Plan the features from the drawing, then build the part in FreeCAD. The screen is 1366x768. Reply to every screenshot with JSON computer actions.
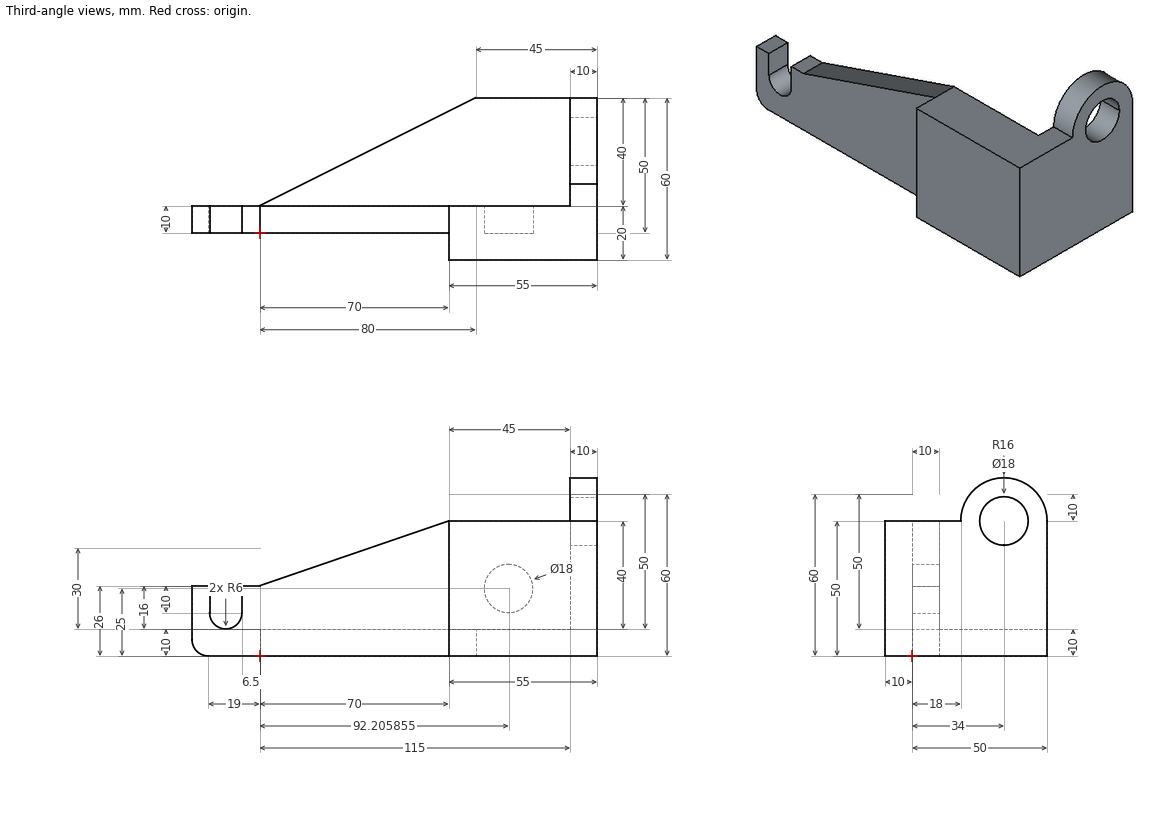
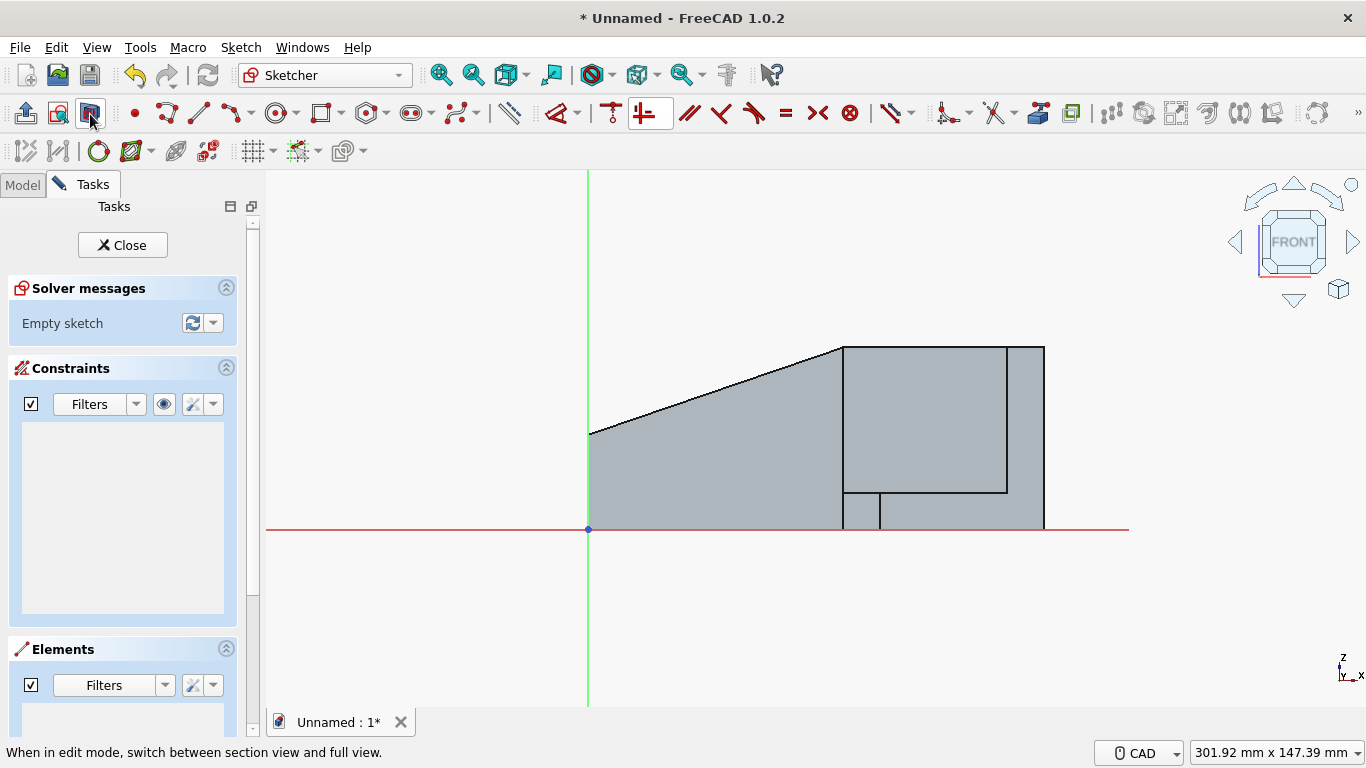
{"action": "scroll", "coordinate": [455, 501], "scroll_direction": "up", "scroll_amount": 6}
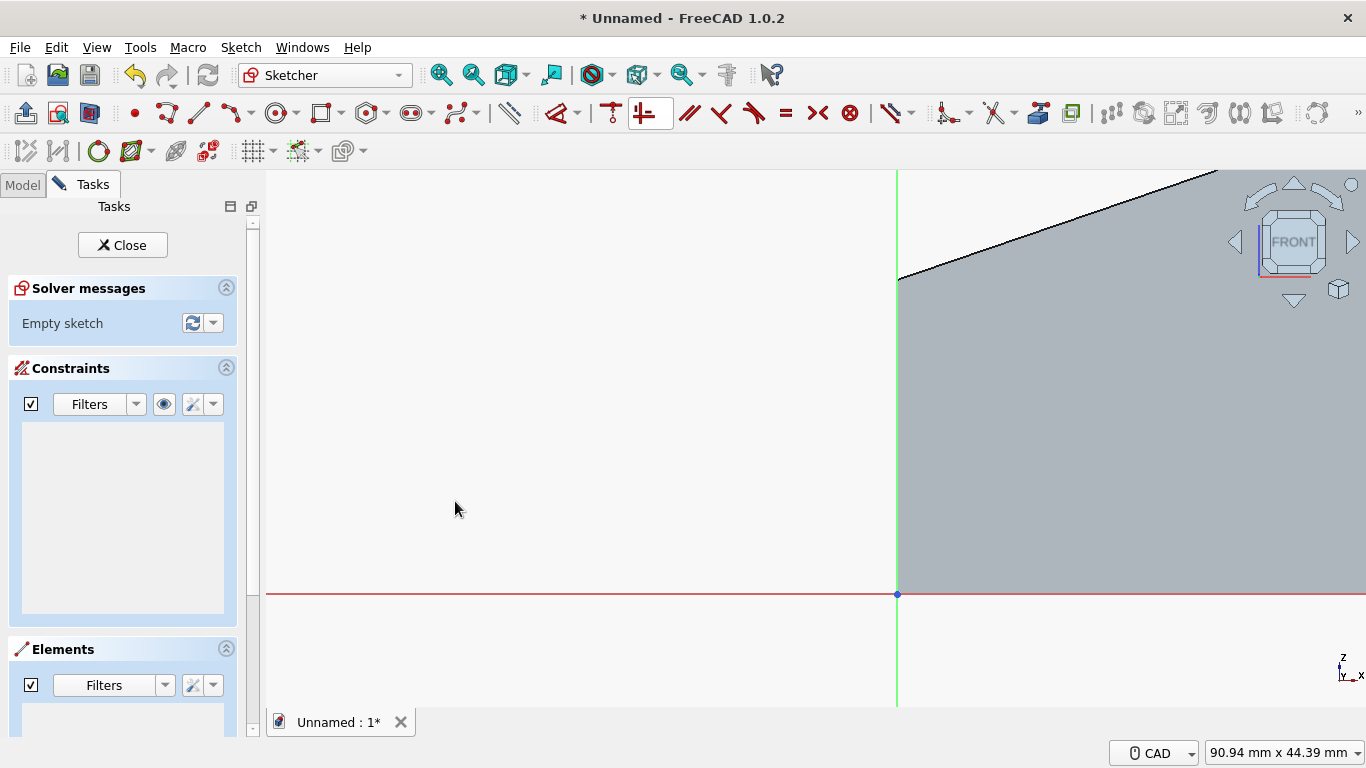
{"action": "left_click", "coordinate": [168, 114]}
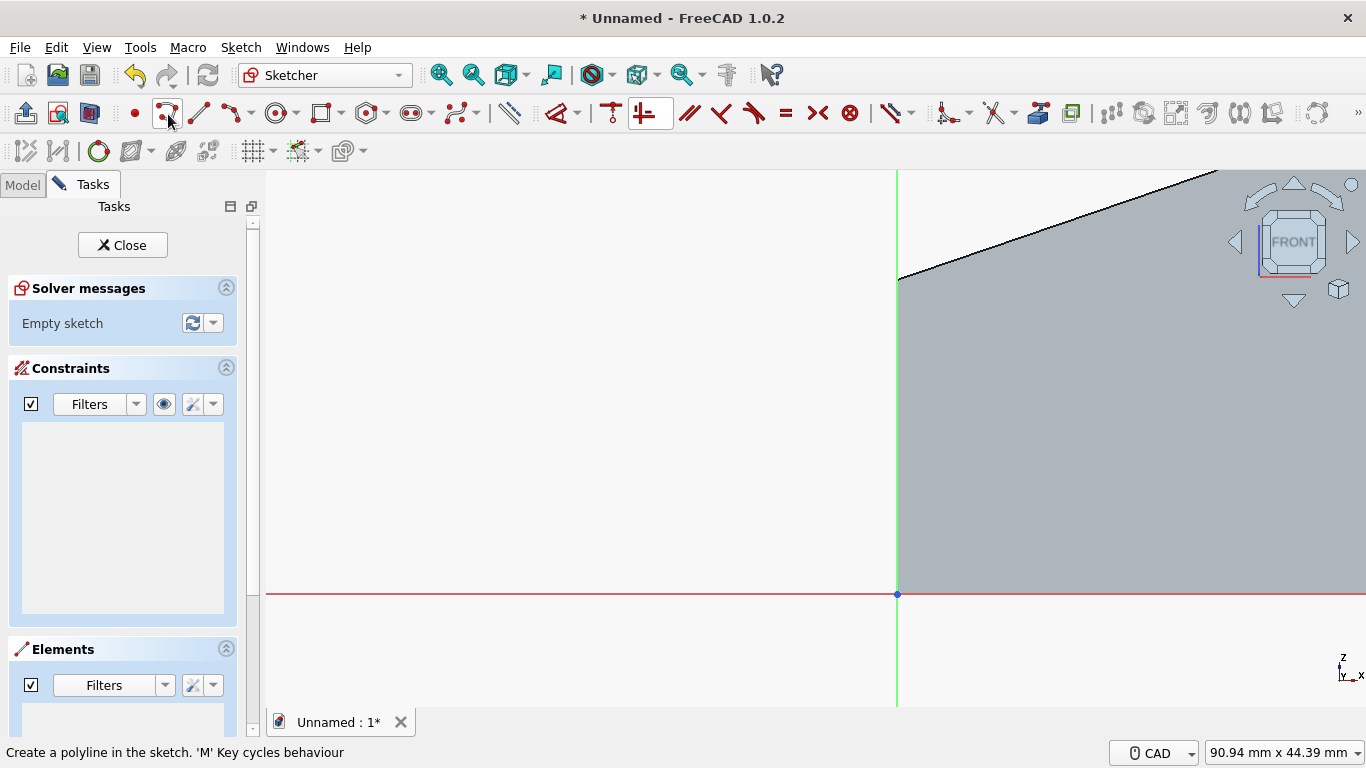
{"action": "left_click", "coordinate": [667, 594]}
{"action": "left_click", "coordinate": [897, 594]}
{"action": "left_click", "coordinate": [888, 280]}
{"action": "left_click", "coordinate": [819, 280]}
{"action": "left_click", "coordinate": [819, 401]}
{"action": "right_click", "coordinate": [819, 401]}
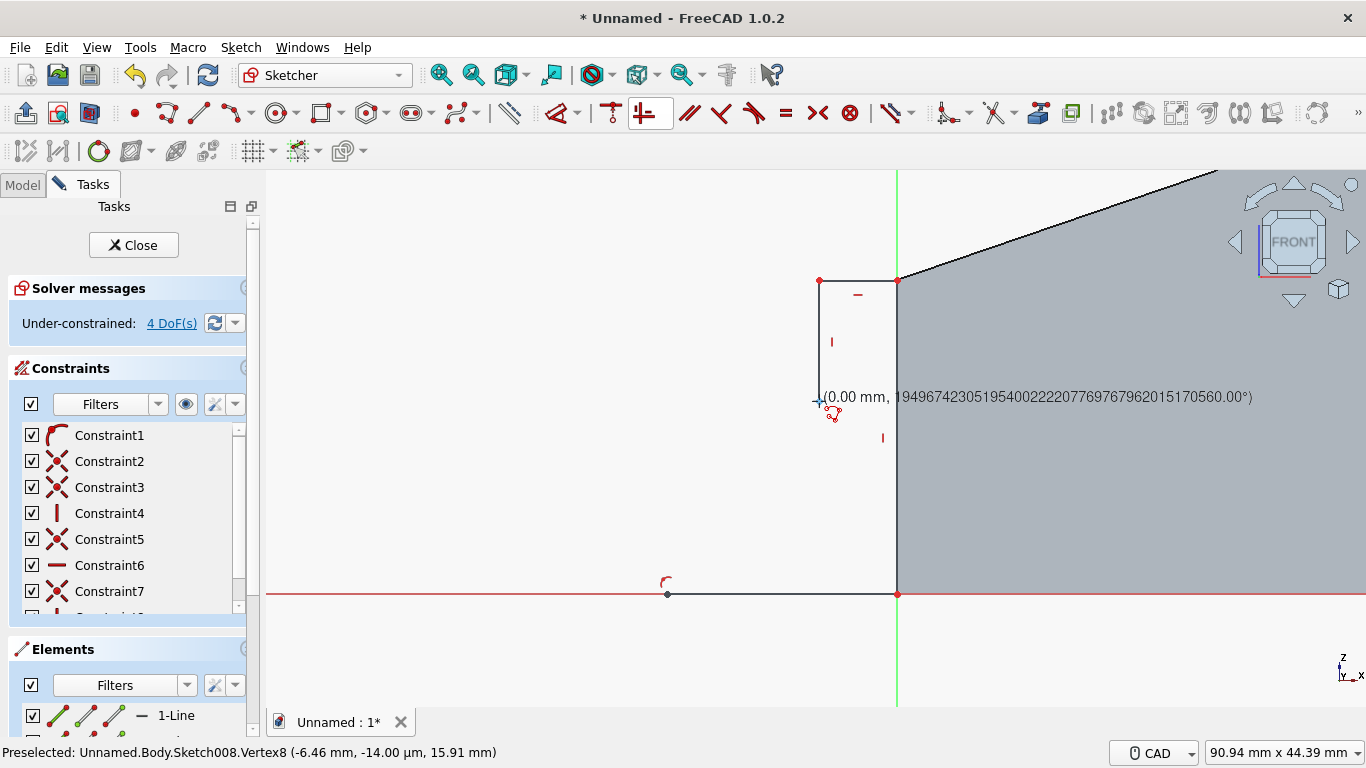
{"action": "left_click", "coordinate": [673, 401]}
{"action": "left_click", "coordinate": [673, 280]}
{"action": "left_click", "coordinate": [595, 280]}
{"action": "left_click", "coordinate": [595, 522]}
{"action": "right_click", "coordinate": [595, 522]}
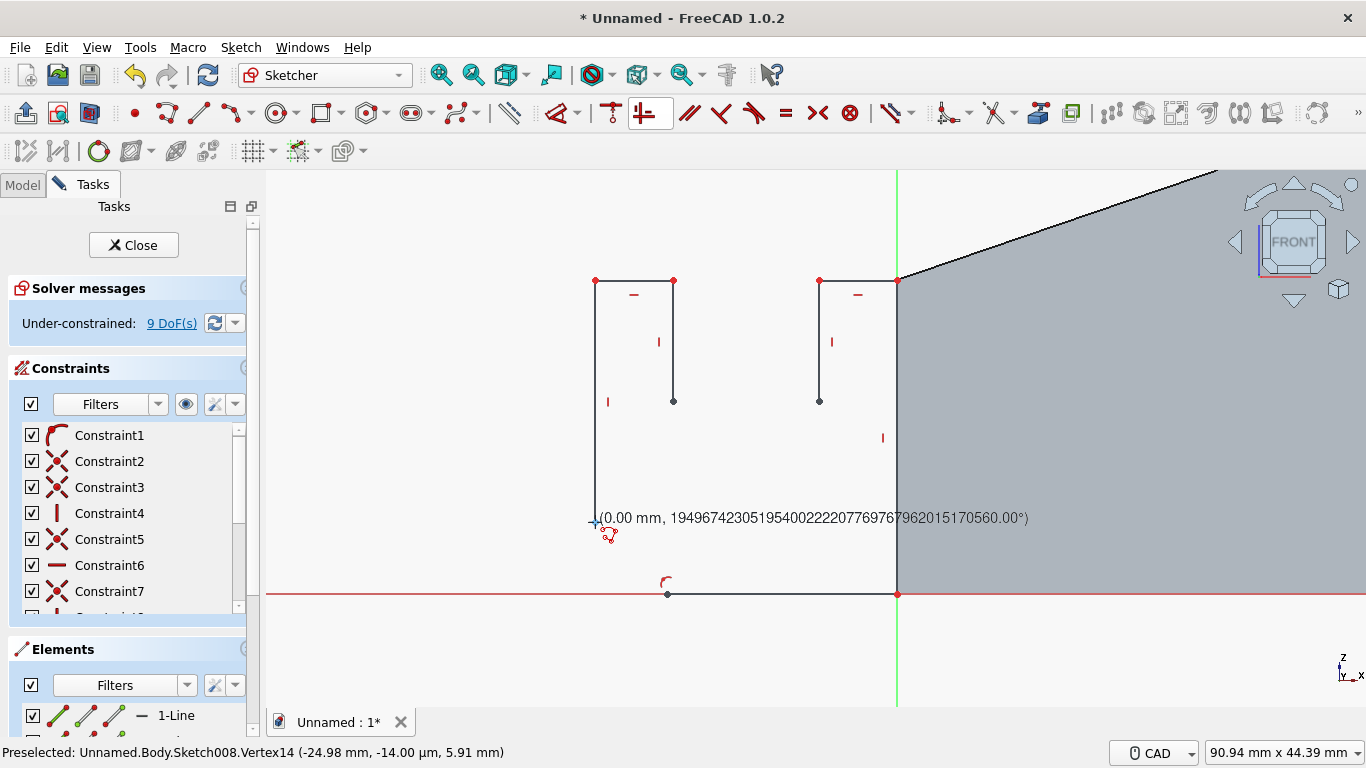
{"action": "left_click", "coordinate": [232, 114]}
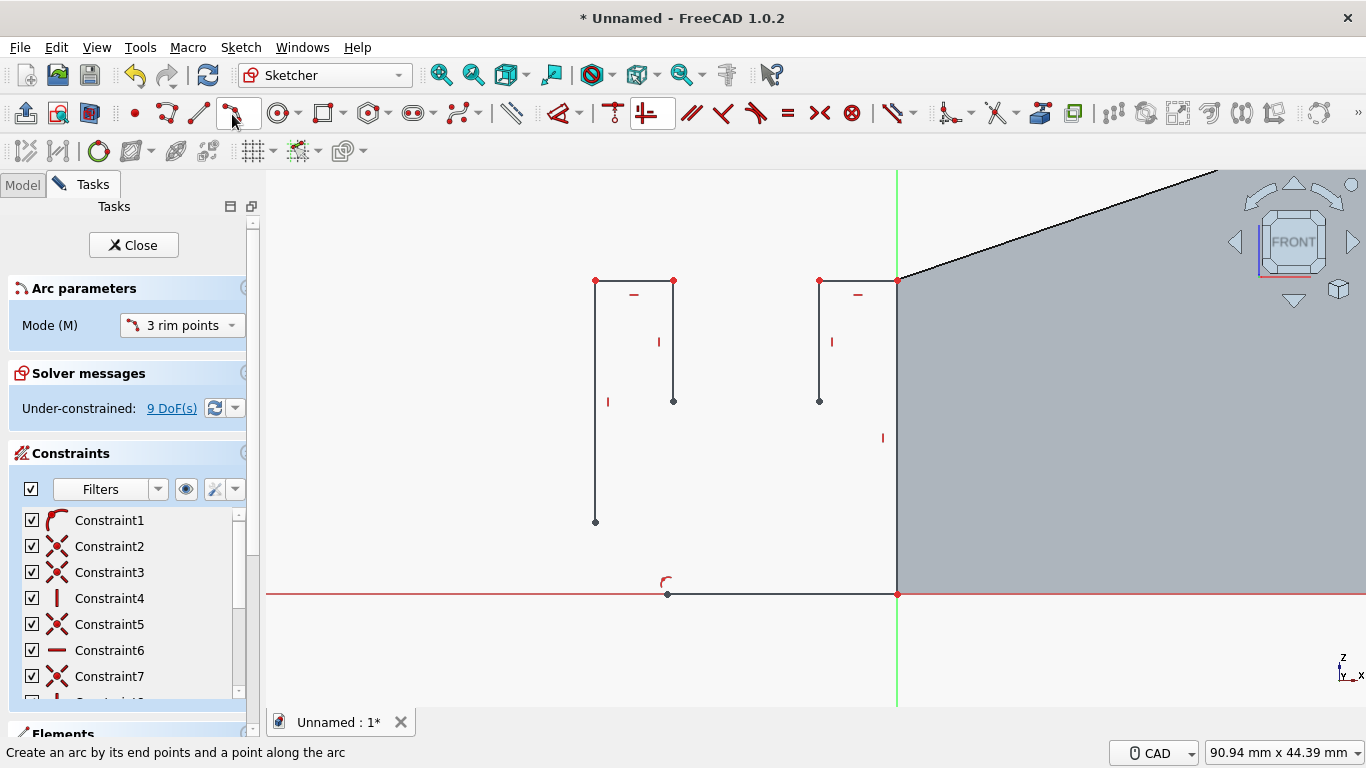
{"action": "left_click", "coordinate": [819, 402]}
{"action": "left_click", "coordinate": [673, 402]}
{"action": "left_click", "coordinate": [746, 474]}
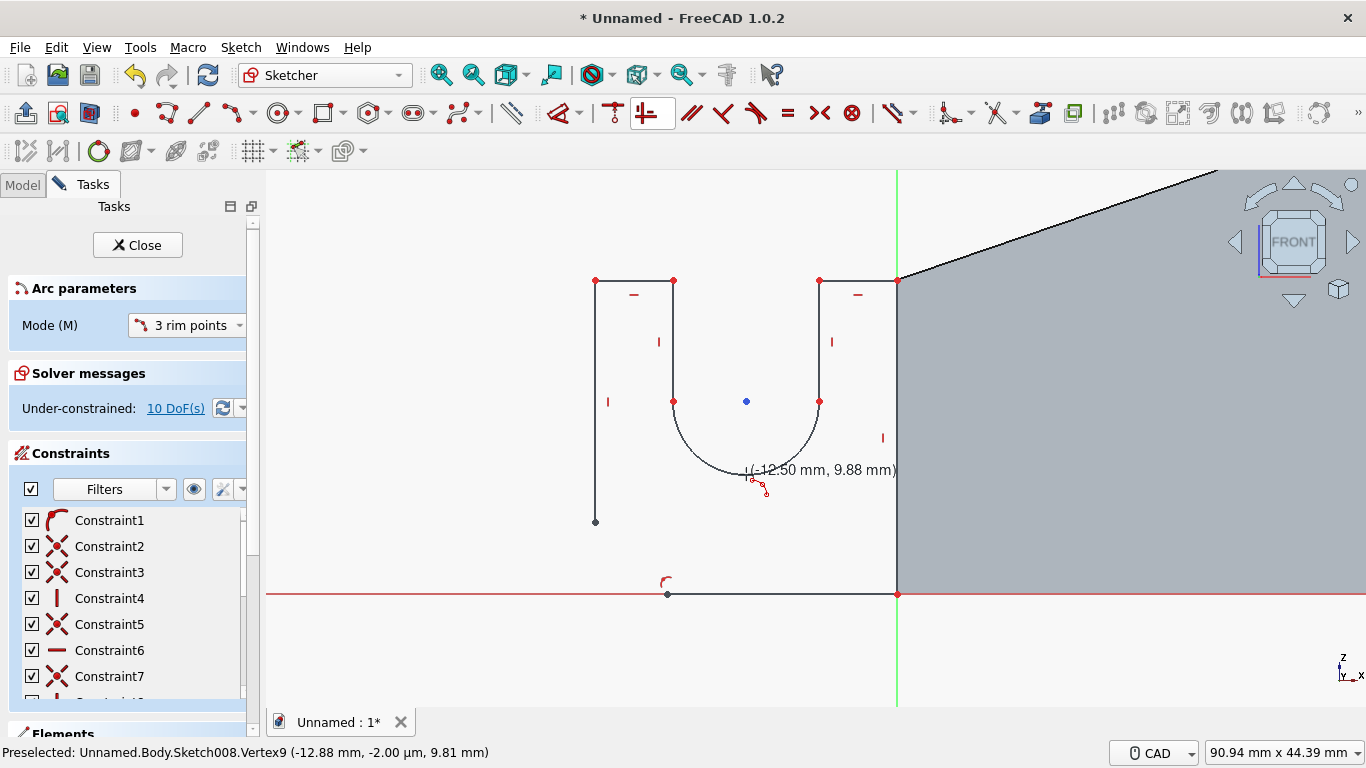
{"action": "left_click", "coordinate": [595, 523]}
{"action": "left_click", "coordinate": [667, 594]}
{"action": "left_click", "coordinate": [616, 573]}
{"action": "key", "text": "Escape"}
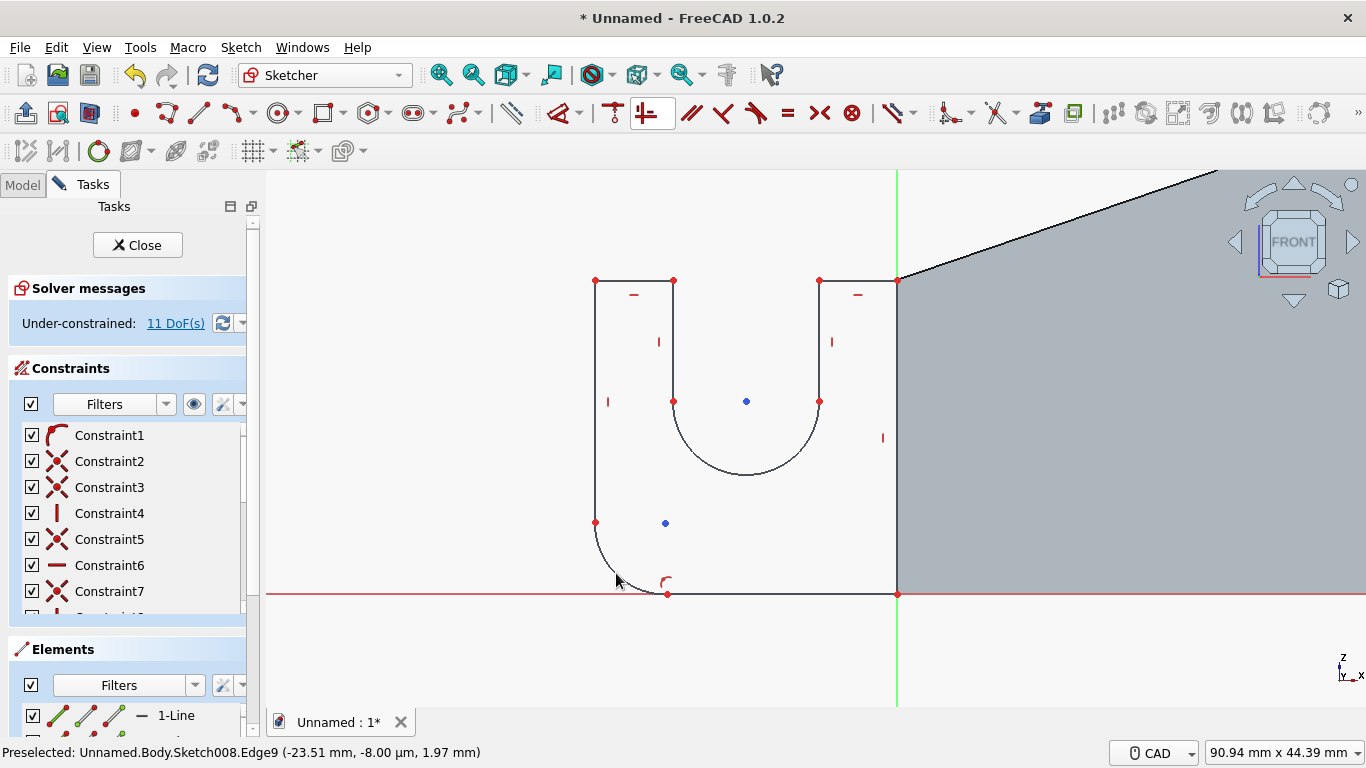
{"action": "left_click", "coordinate": [736, 594]}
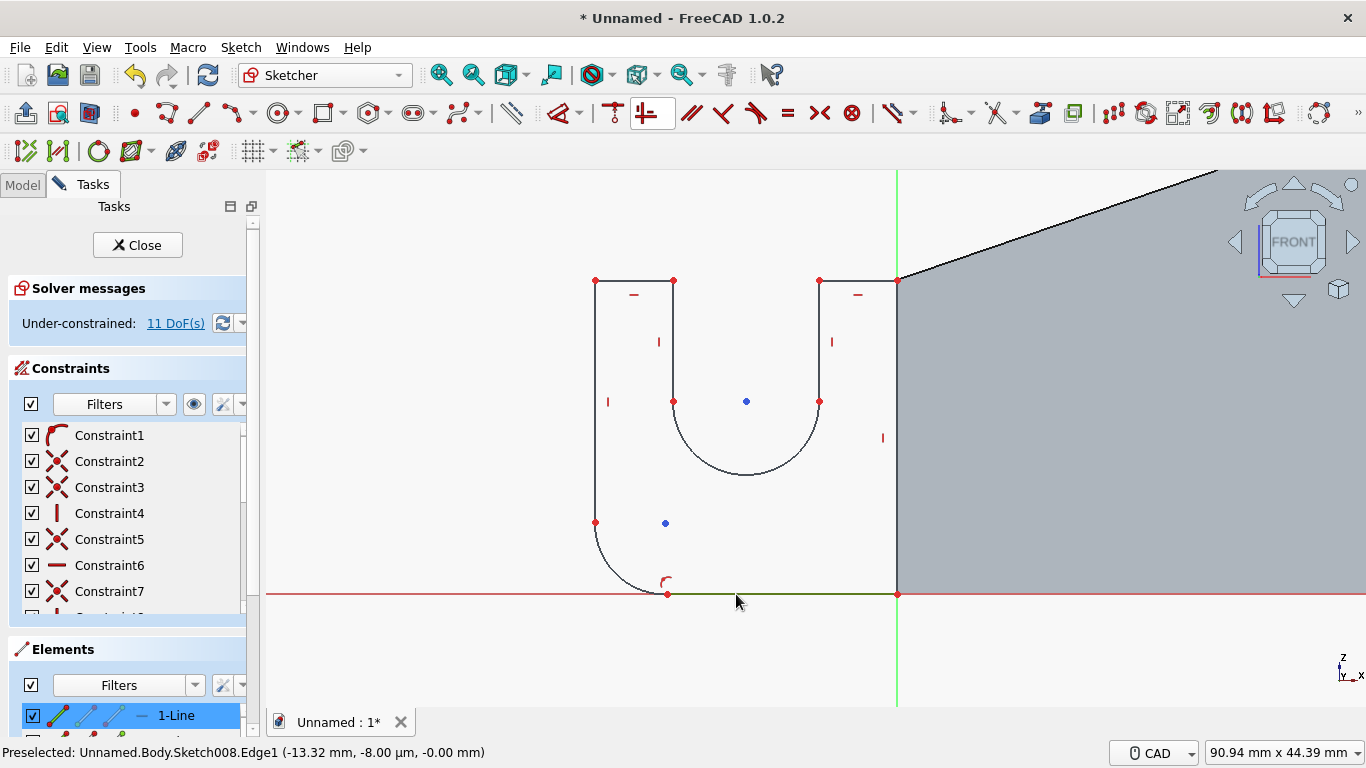
{"action": "left_click", "coordinate": [603, 556]}